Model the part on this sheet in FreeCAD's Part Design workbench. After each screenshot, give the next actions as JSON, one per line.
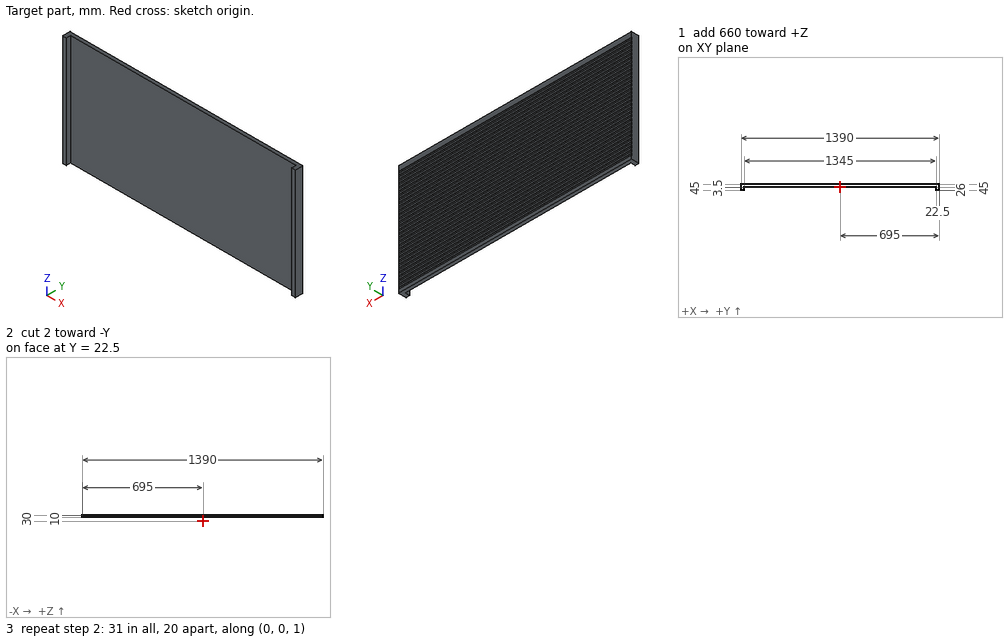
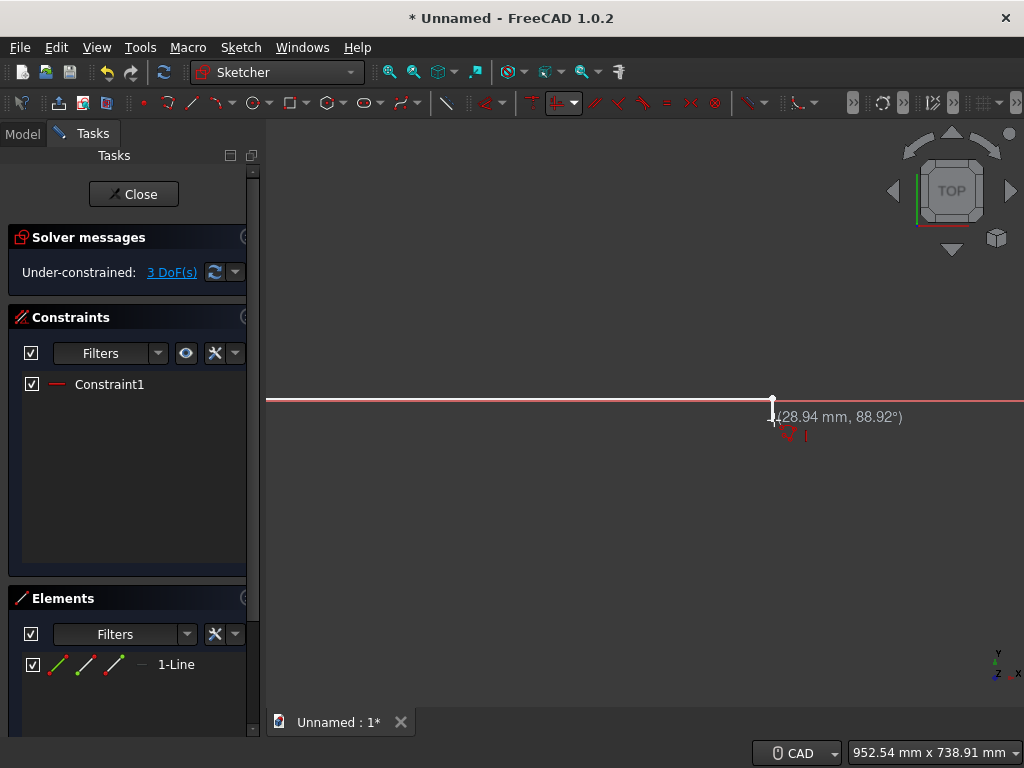
{"action": "left_click", "coordinate": [772, 419]}
{"action": "left_click", "coordinate": [790, 419]}
{"action": "left_click", "coordinate": [790, 383]}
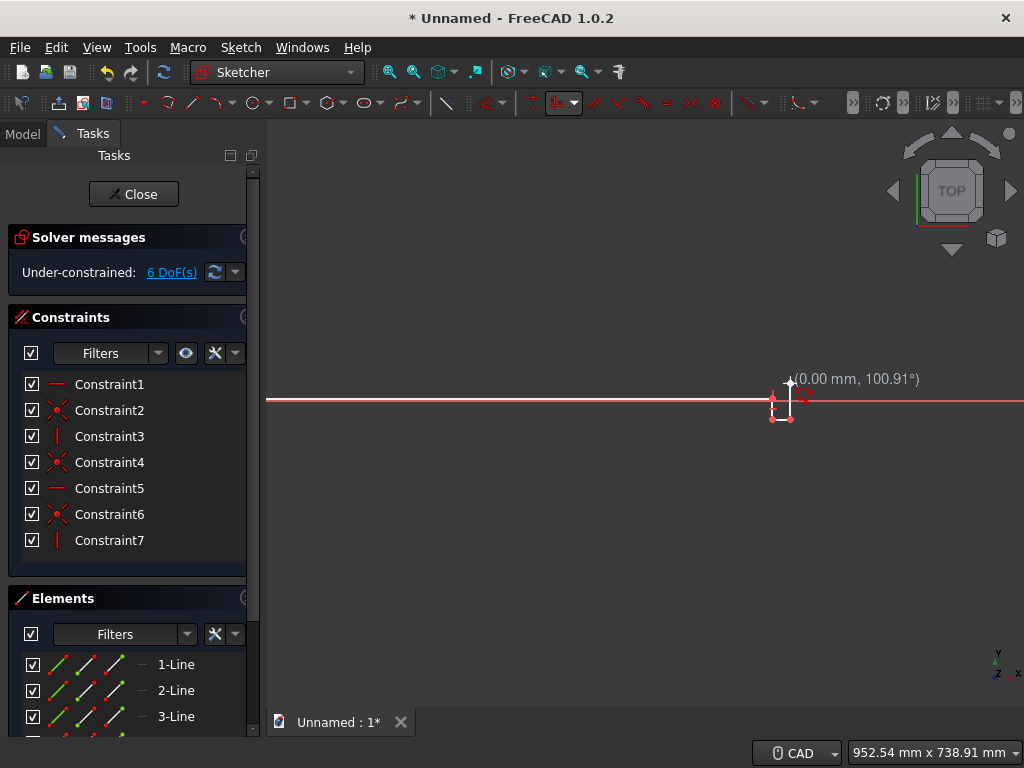
{"action": "scroll", "coordinate": [774, 420], "scroll_direction": "down", "scroll_amount": 5}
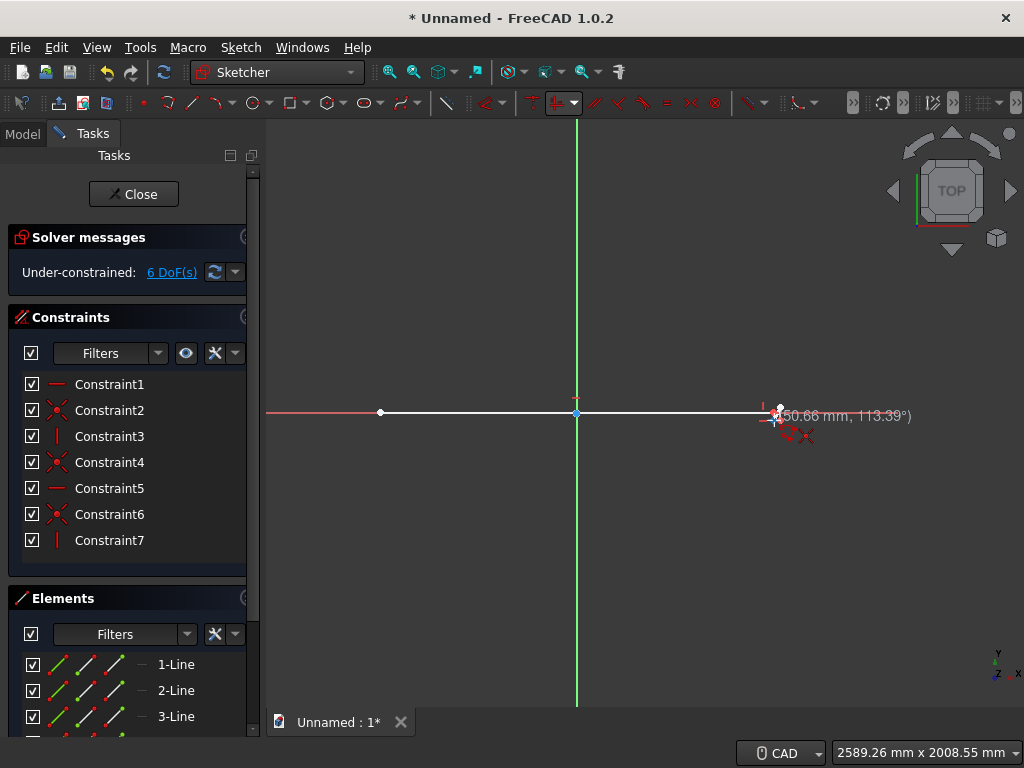
{"action": "scroll", "coordinate": [374, 407], "scroll_direction": "up", "scroll_amount": 5}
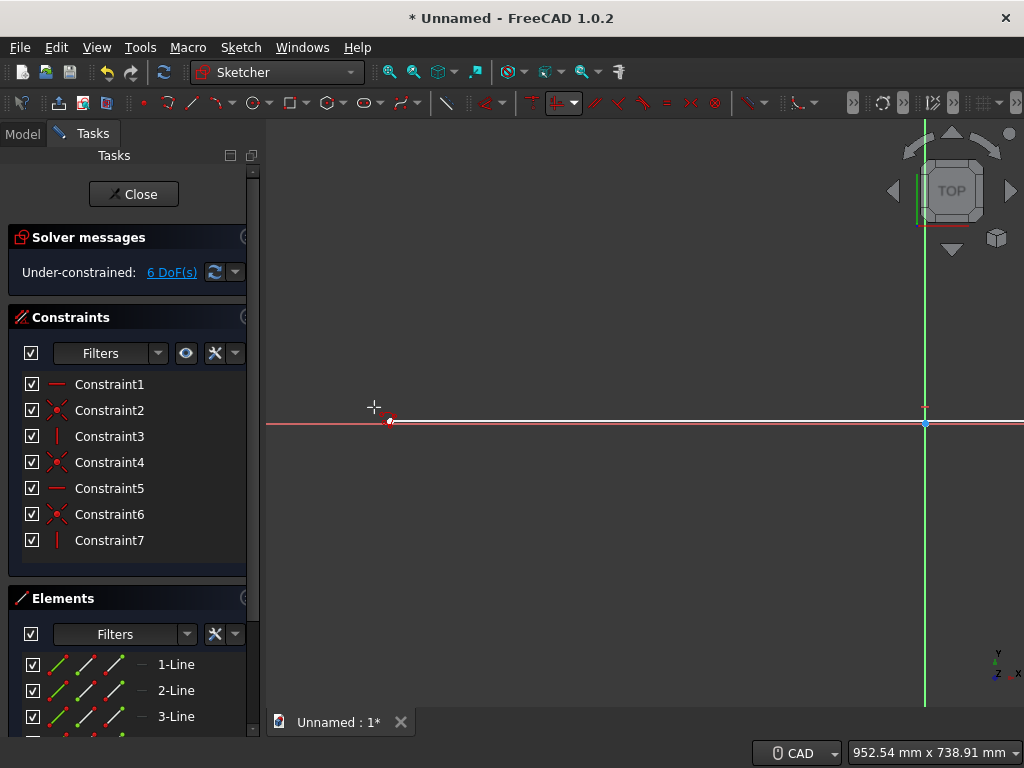
{"action": "left_click", "coordinate": [372, 405]}
{"action": "left_click", "coordinate": [372, 442]}
{"action": "left_click", "coordinate": [390, 442]}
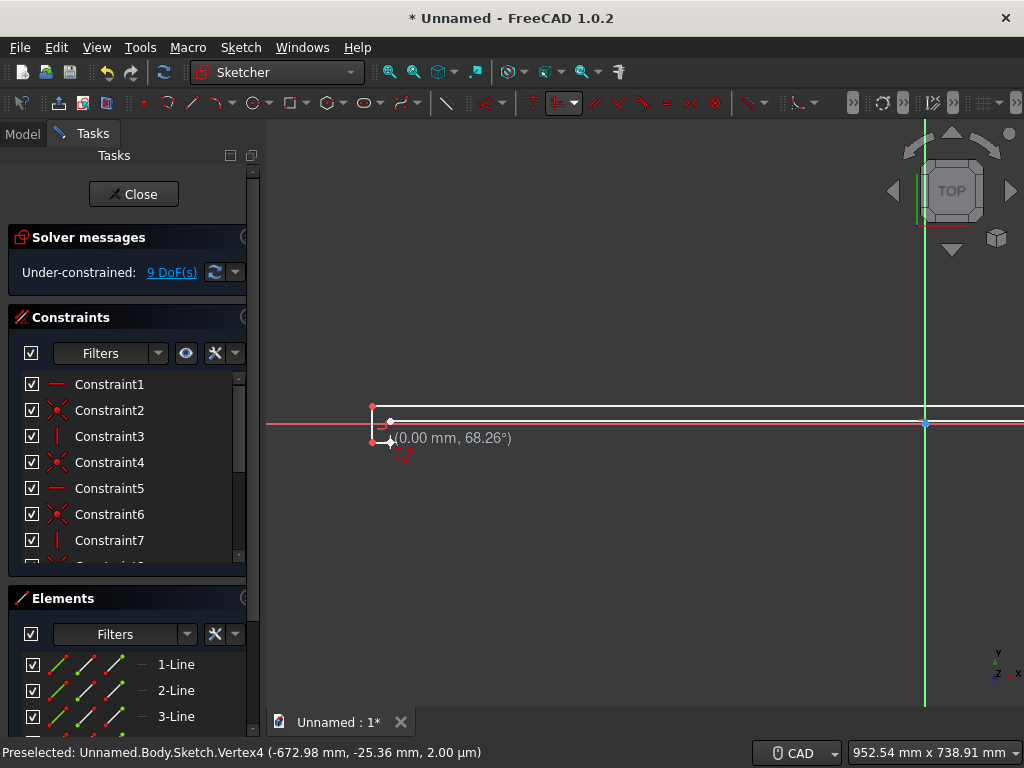
{"action": "scroll", "coordinate": [390, 421], "scroll_direction": "up", "scroll_amount": 9}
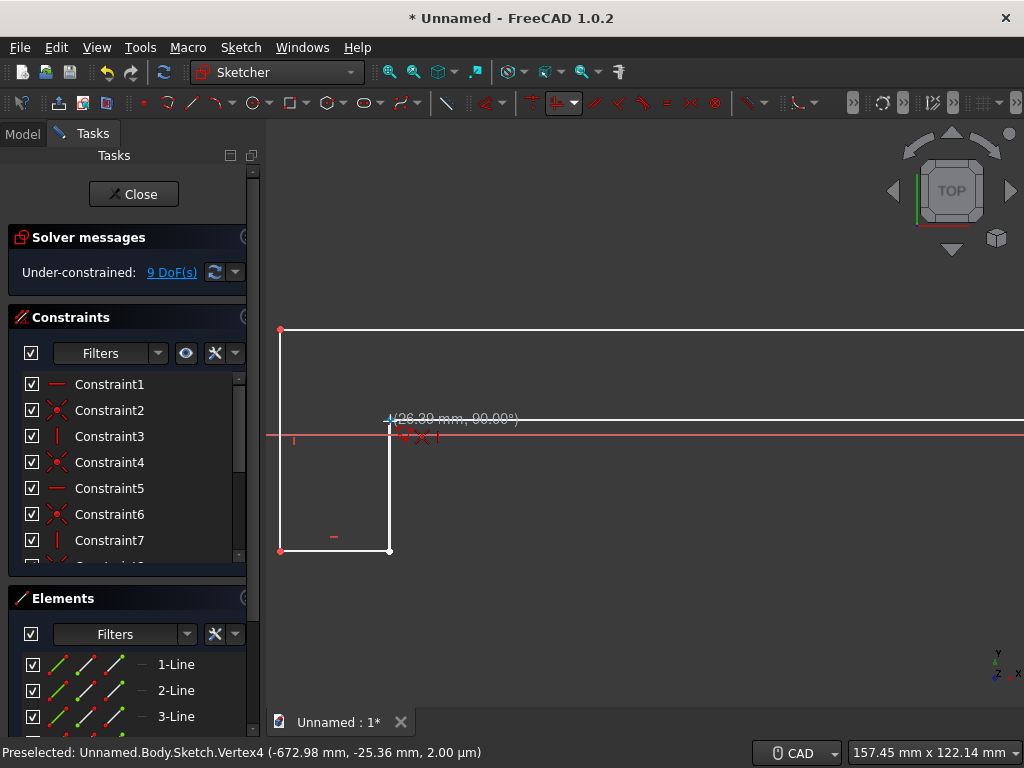
{"action": "left_click", "coordinate": [391, 420]}
{"action": "key", "text": "Escape"}
{"action": "key", "text": "Escape"}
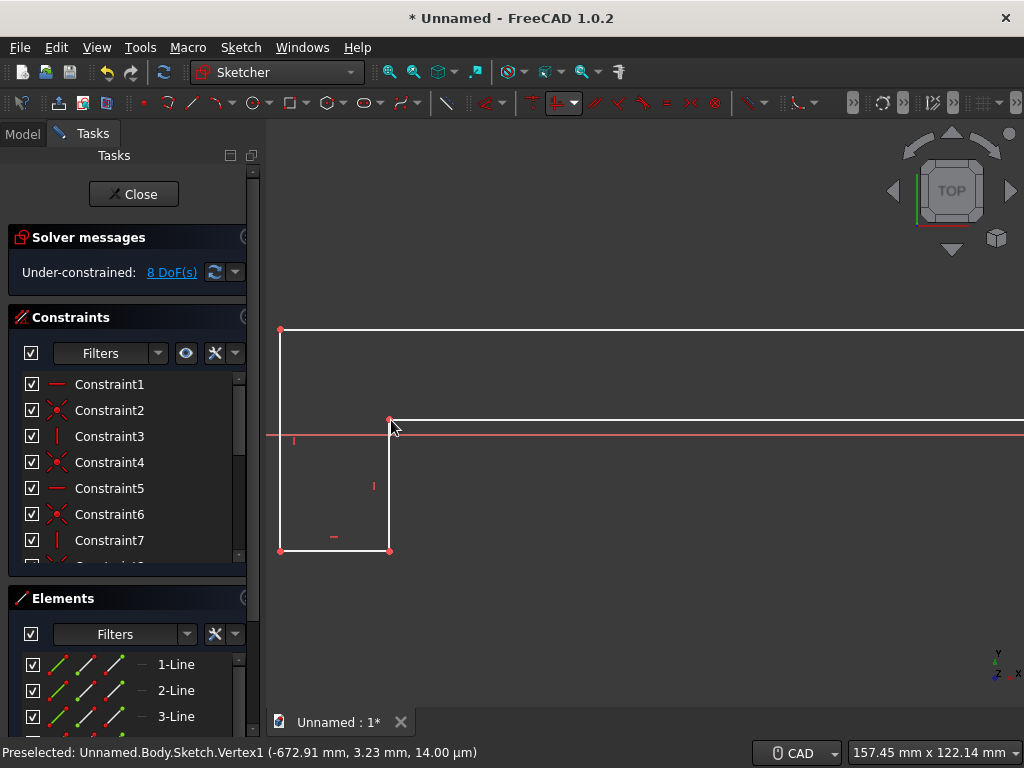
{"action": "key", "text": "d"}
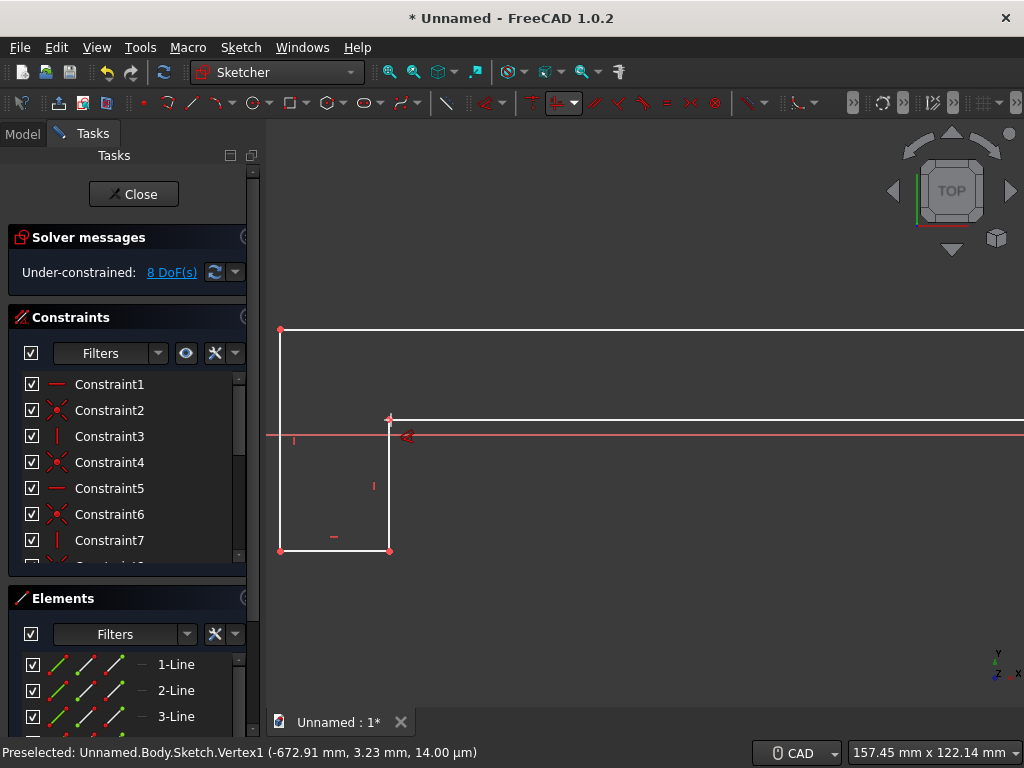
{"action": "scroll", "coordinate": [379, 412], "scroll_direction": "down", "scroll_amount": 14}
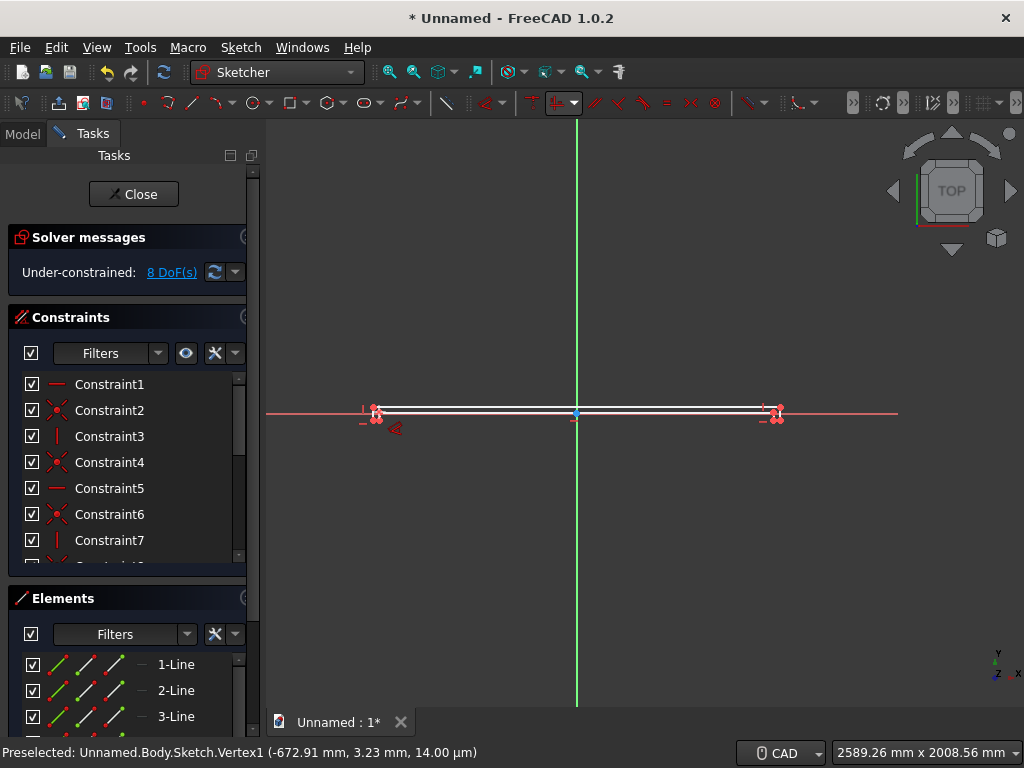
{"action": "scroll", "coordinate": [774, 415], "scroll_direction": "up", "scroll_amount": 12}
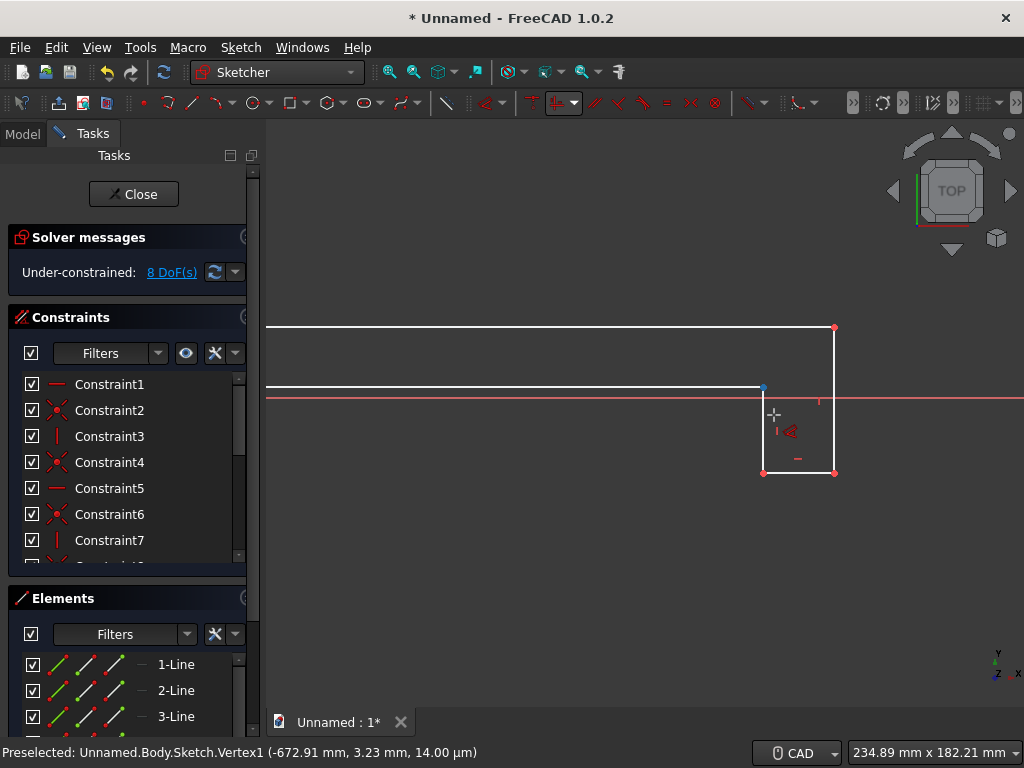
{"action": "left_click", "coordinate": [763, 413]}
{"action": "left_click", "coordinate": [797, 430]}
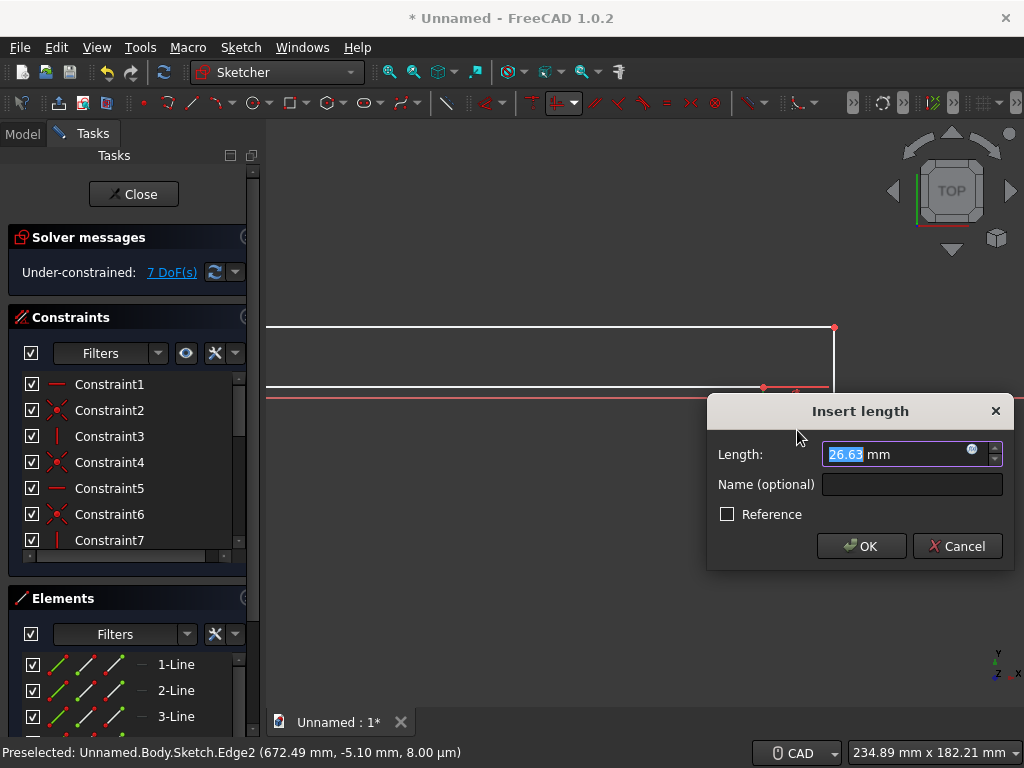
{"action": "type", "text": "26"}
{"action": "key", "text": "Return"}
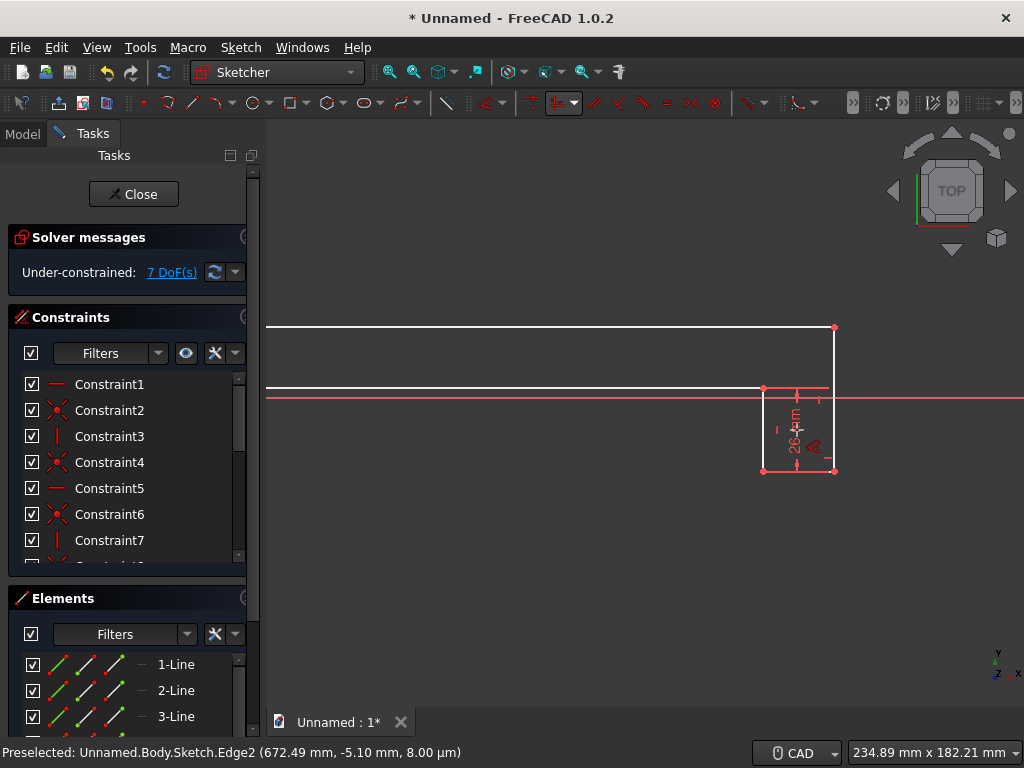
{"action": "left_click", "coordinate": [834, 428]}
{"action": "left_click", "coordinate": [800, 366]}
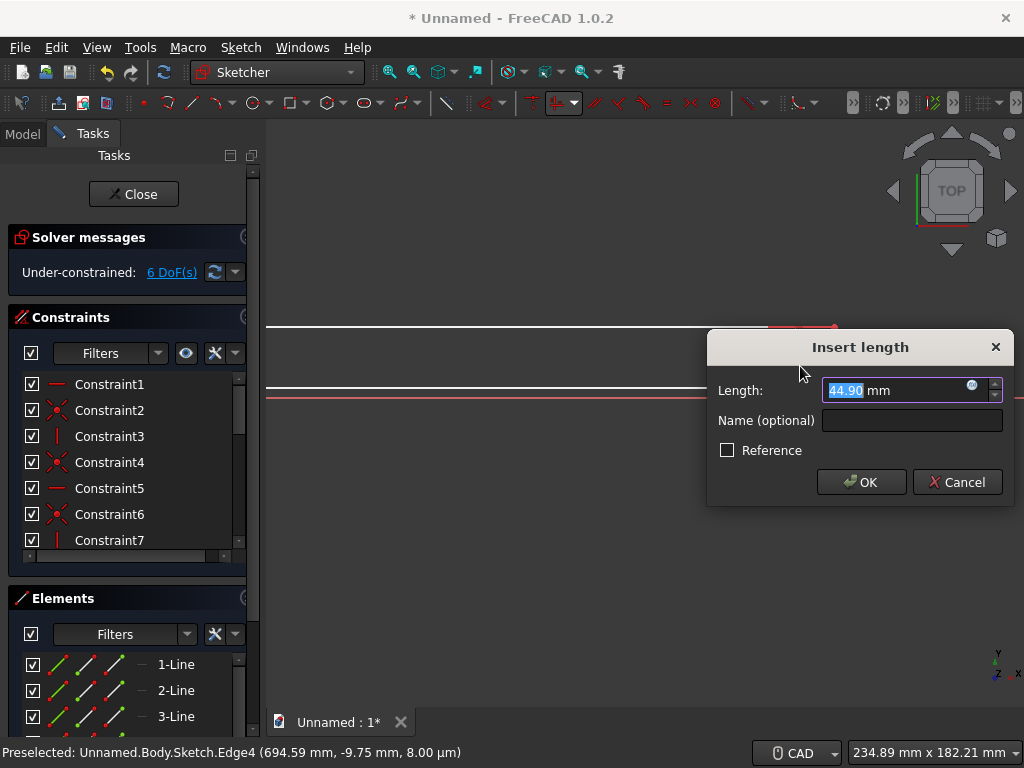
{"action": "type", "text": "45"}
{"action": "key", "text": "Return"}